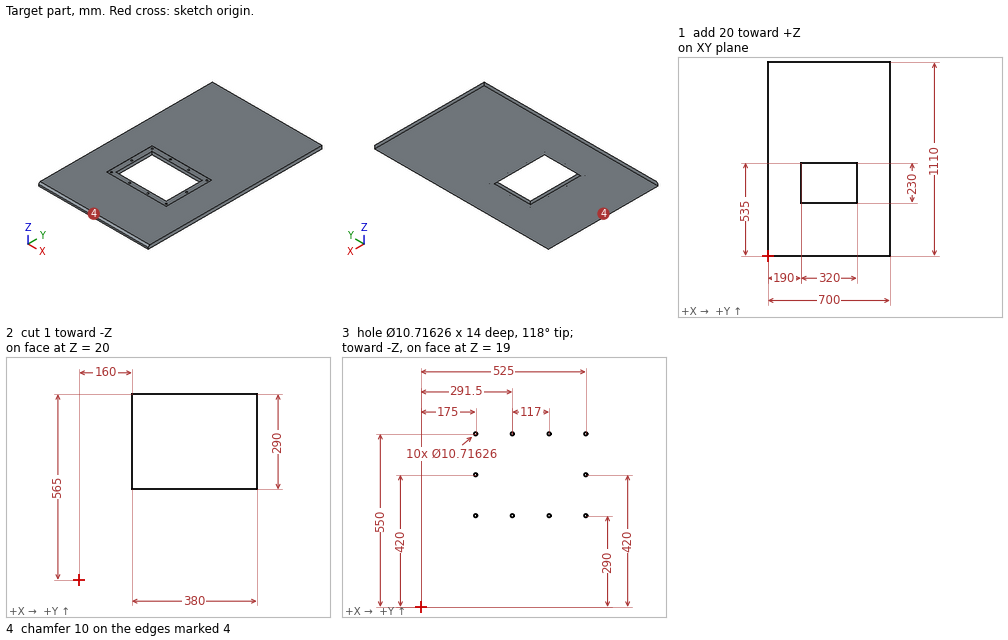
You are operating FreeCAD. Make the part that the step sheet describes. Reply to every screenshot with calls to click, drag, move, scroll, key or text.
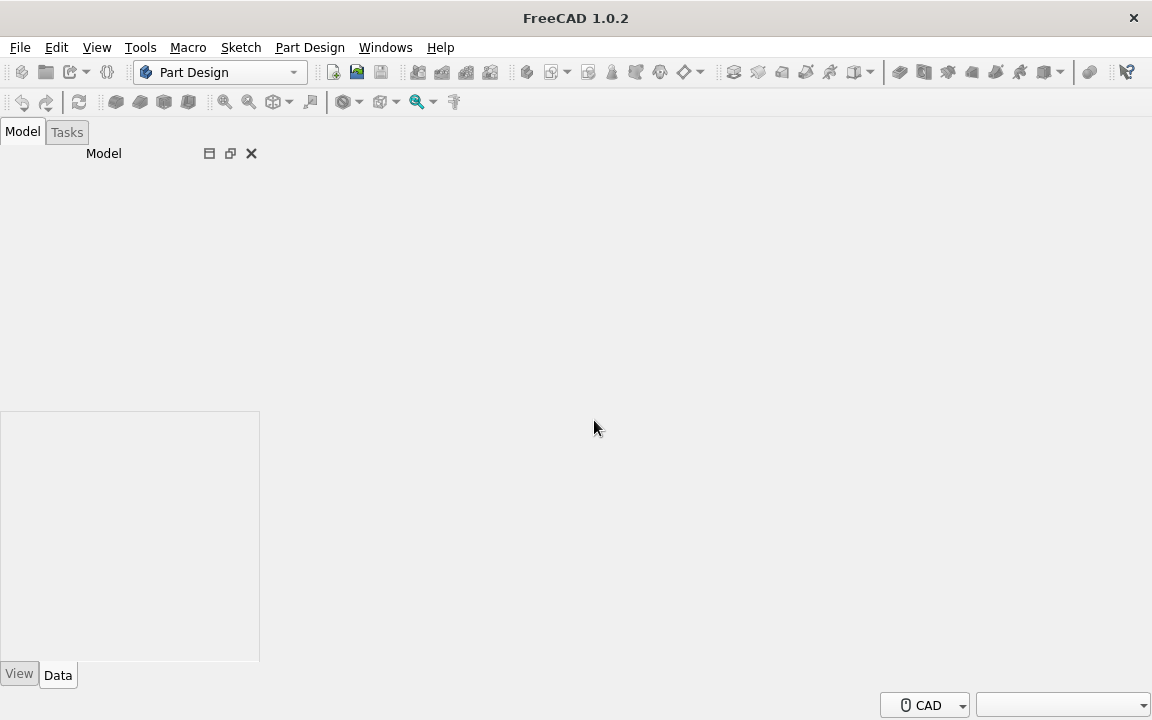
key(ctrl+n)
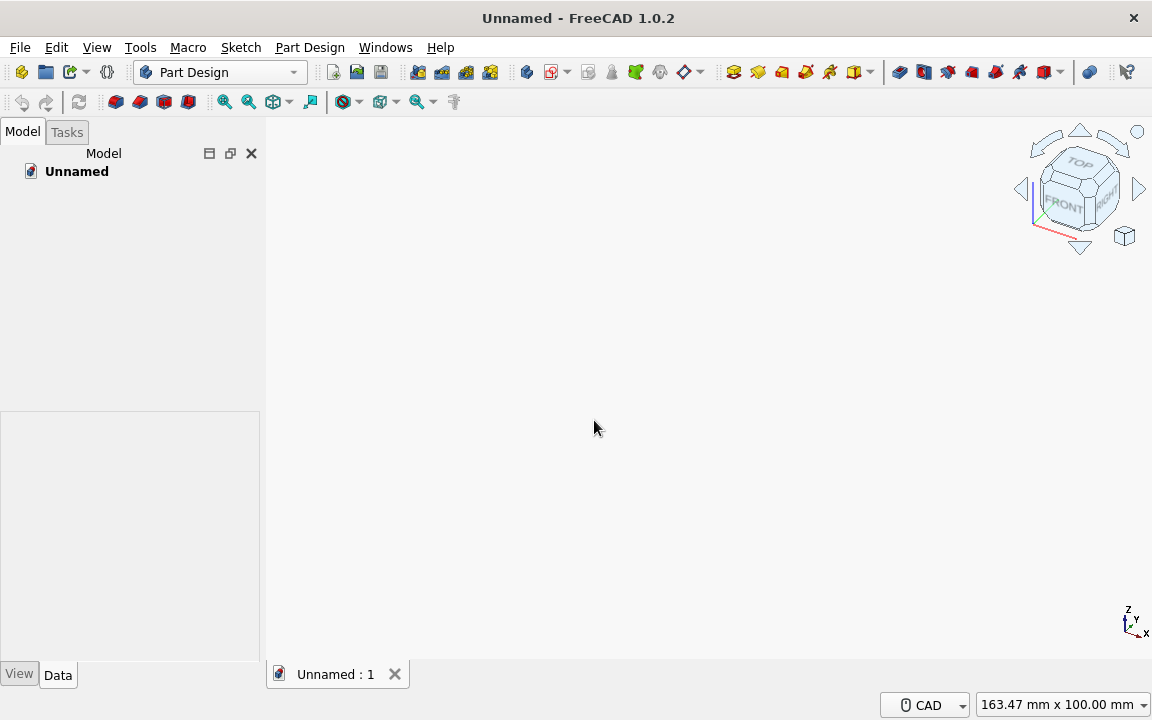
click(552, 72)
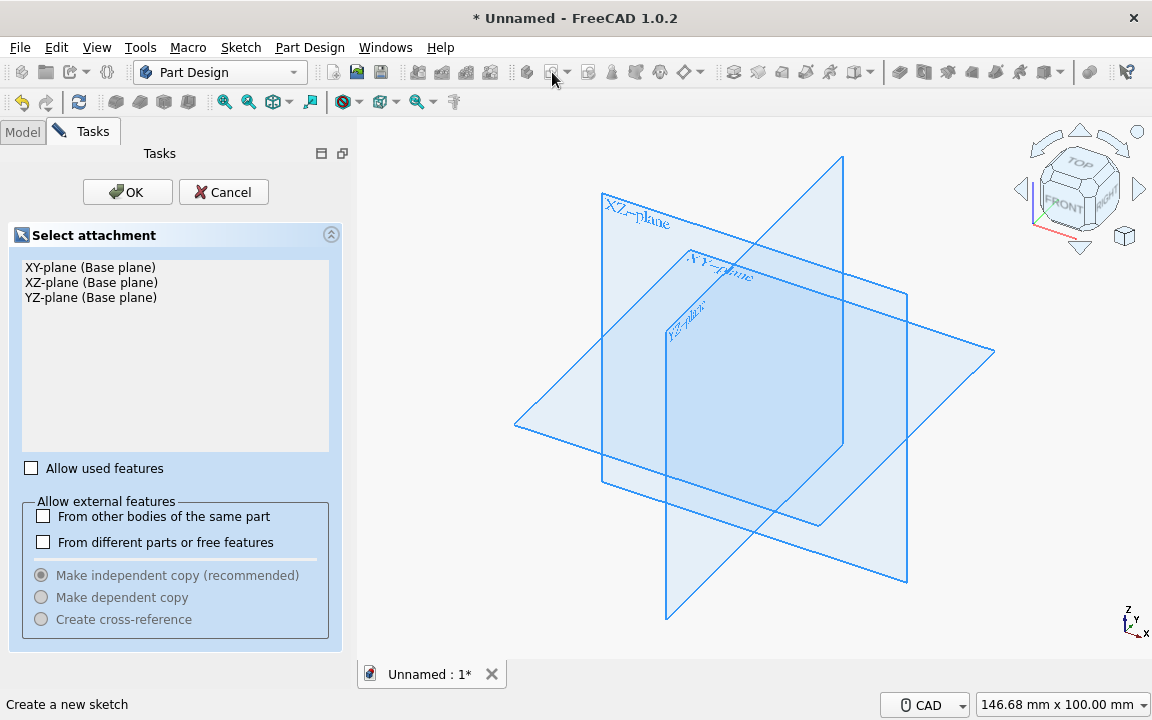
click(82, 268)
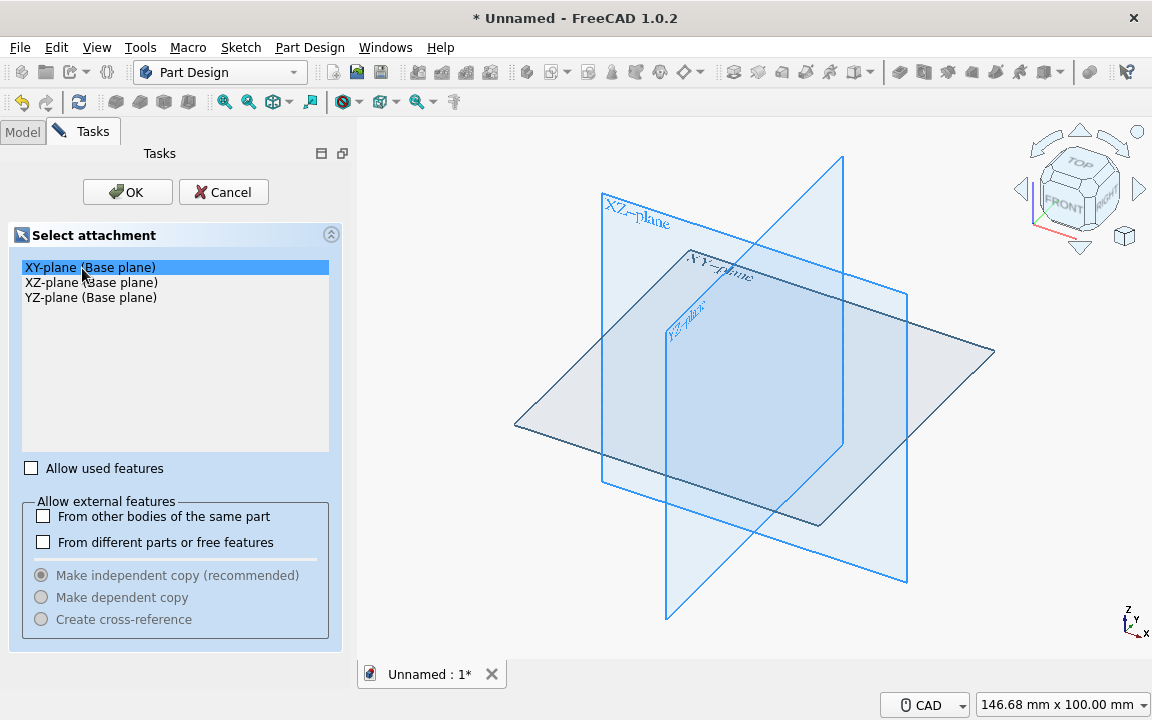
click(128, 192)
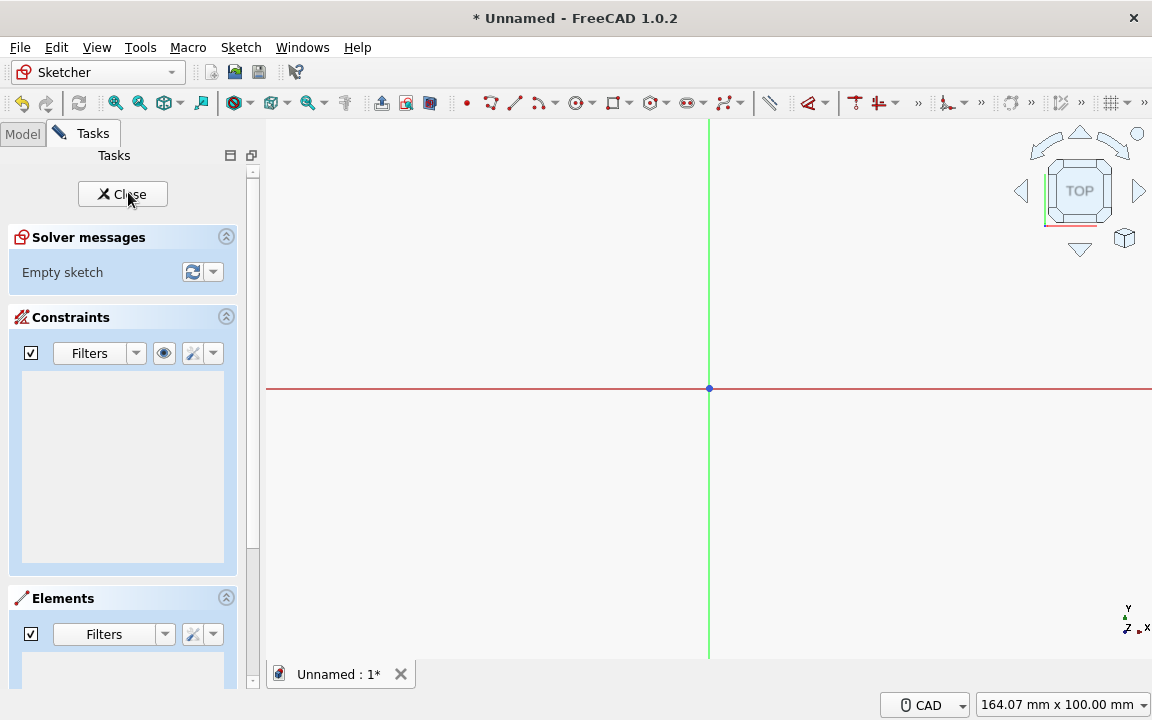
scroll(514, 583, down, 14)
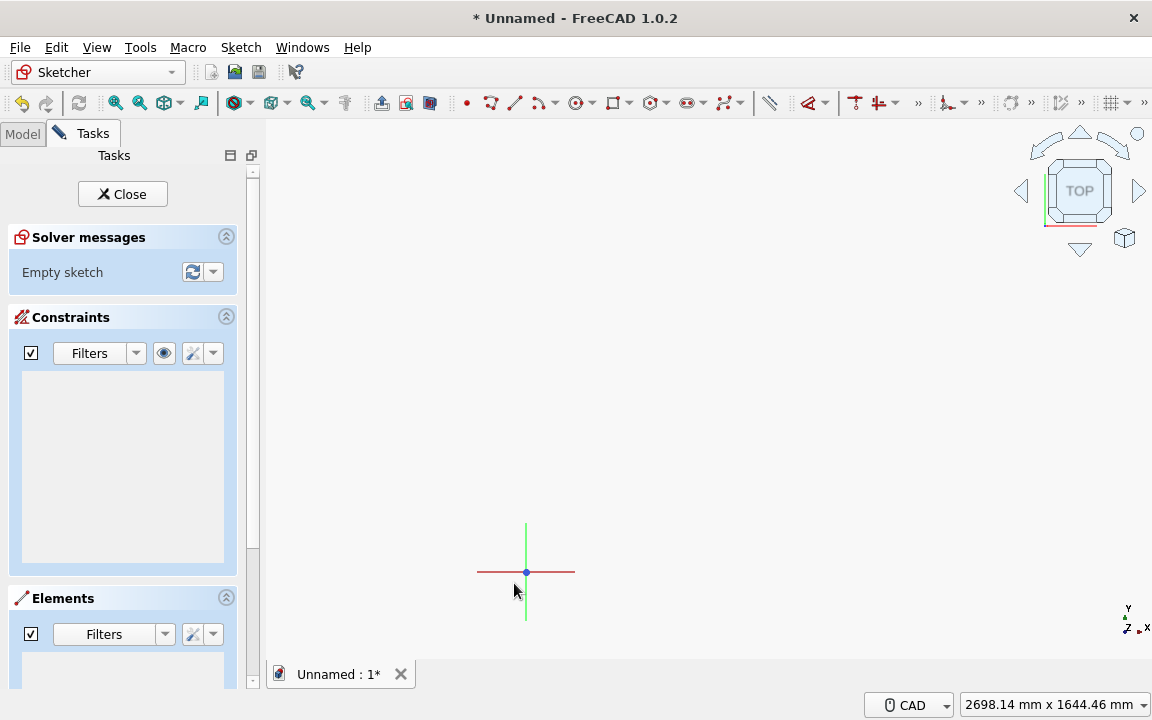
key(g)
key(r)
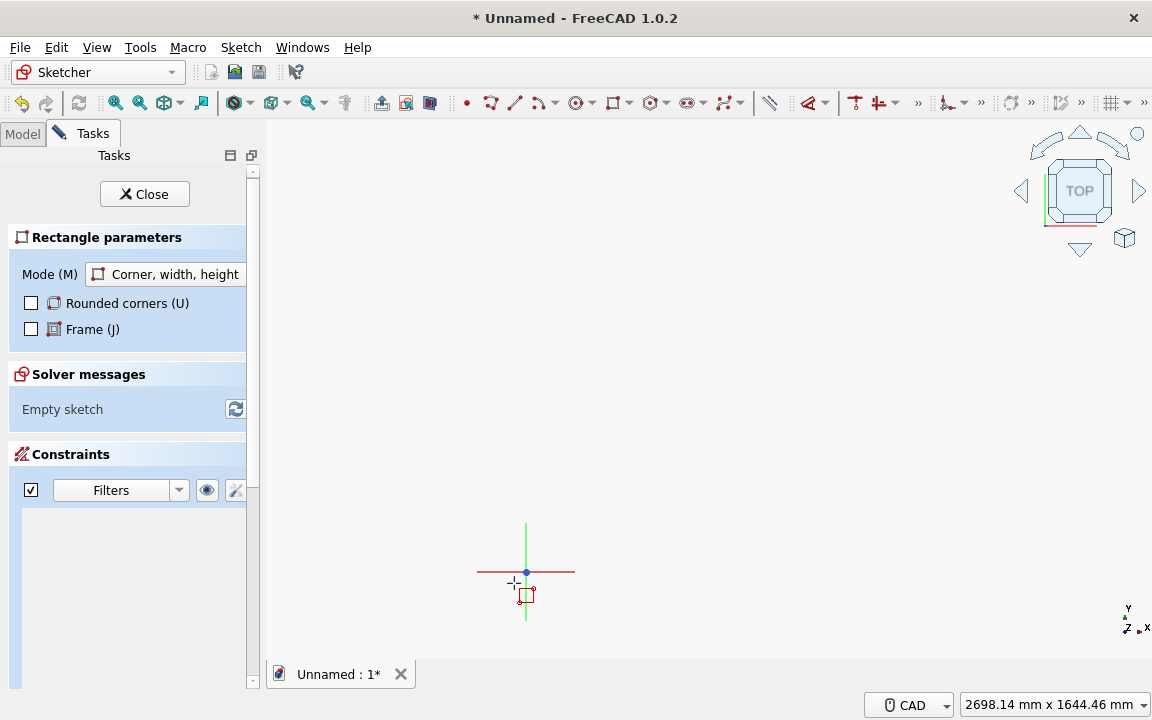
click(526, 572)
move(756, 208)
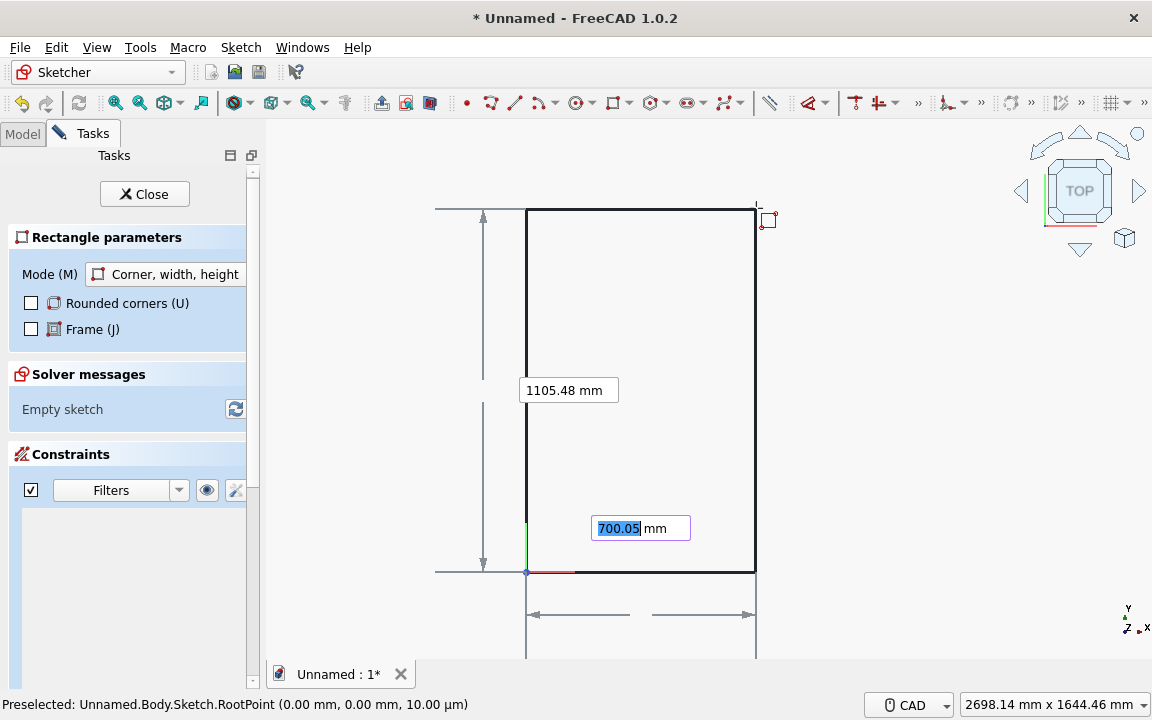
text(700)
key(Tab)
text(1110)
key(Return)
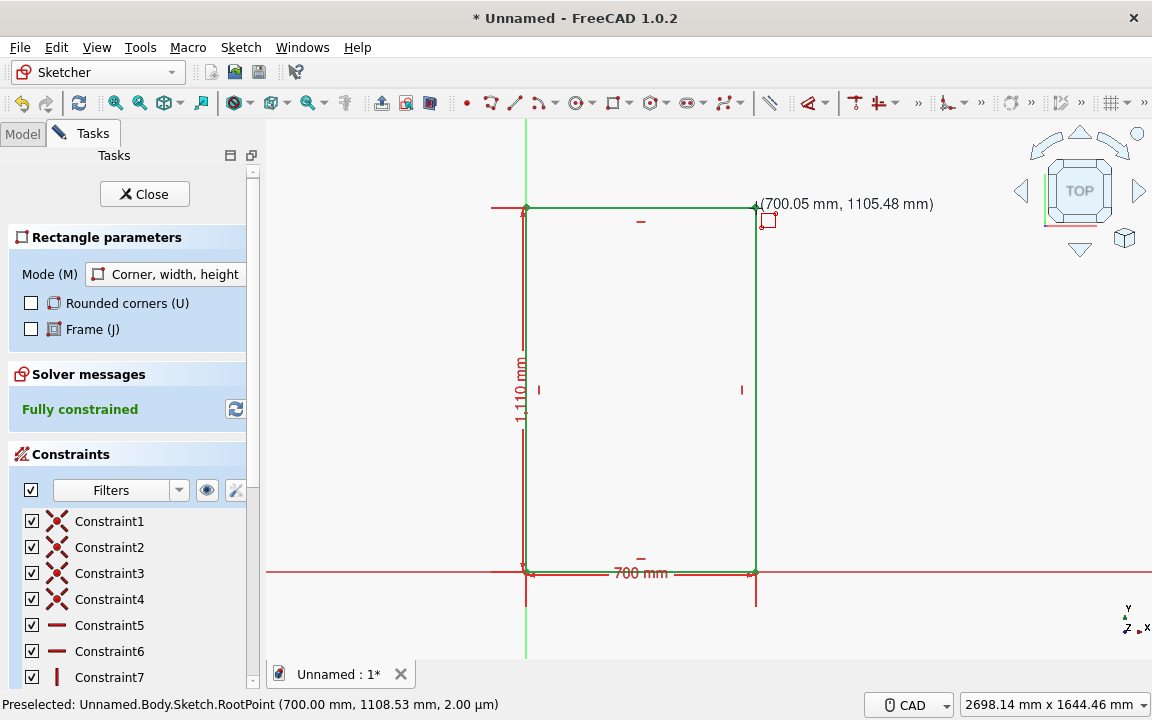
click(589, 396)
move(694, 472)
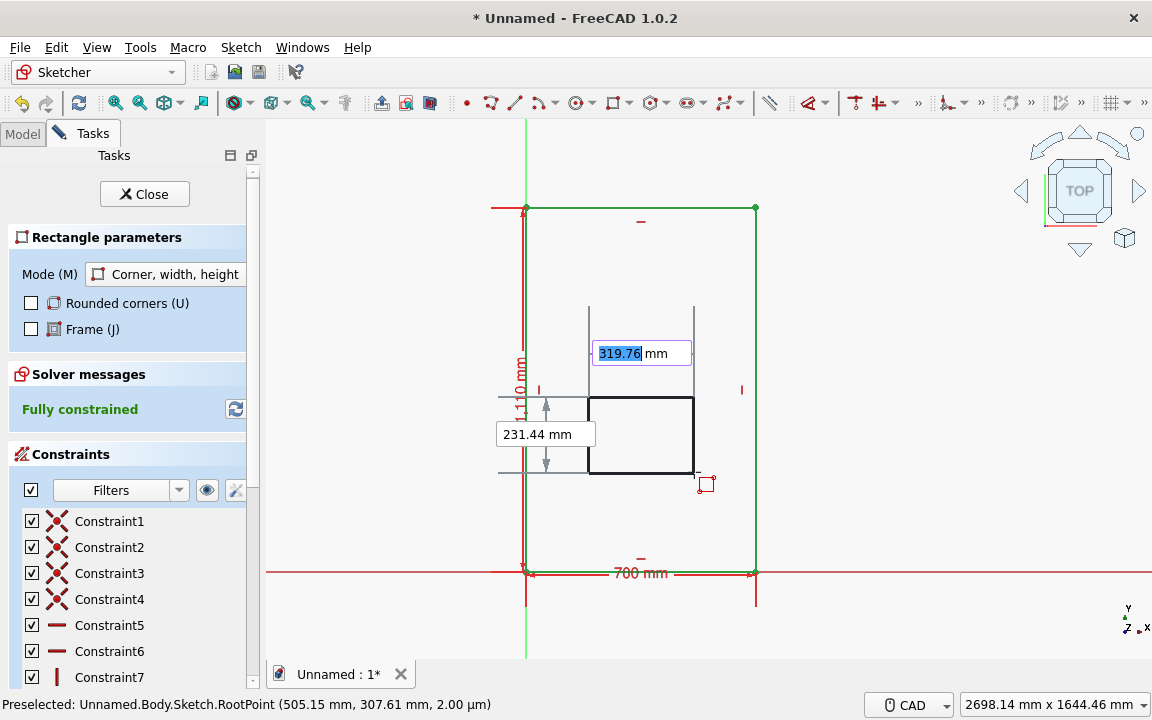
text(320)
key(Tab)
text(230)
key(Return)
key(Escape)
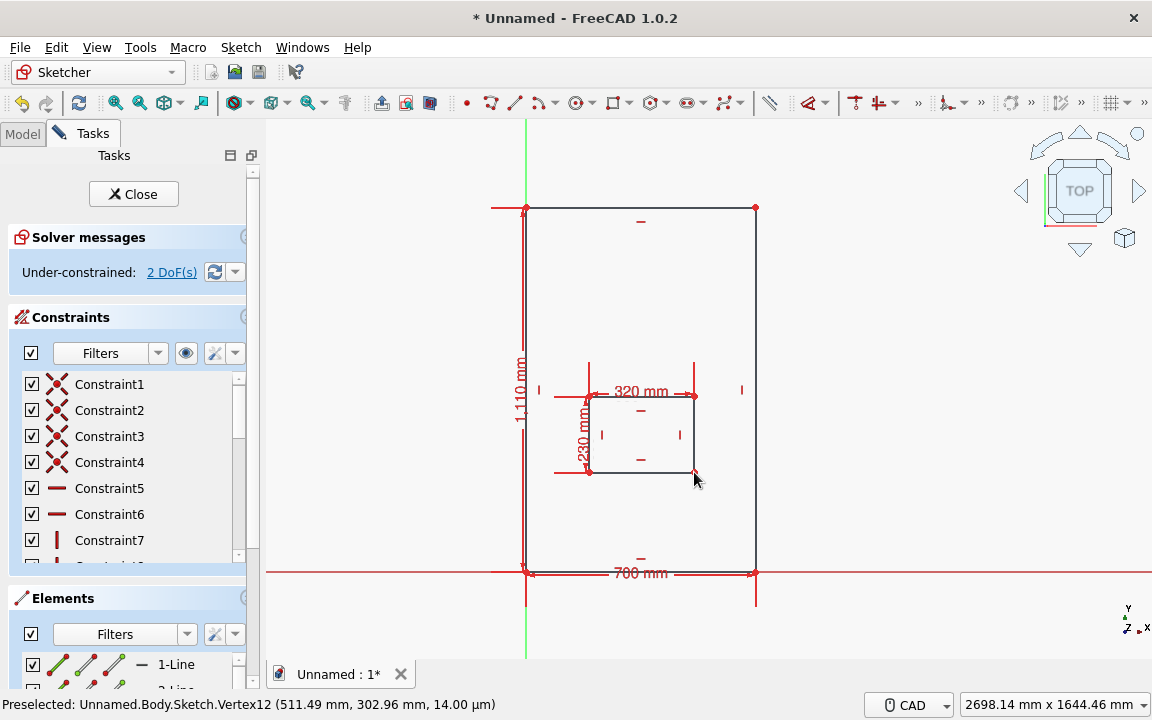
key(d)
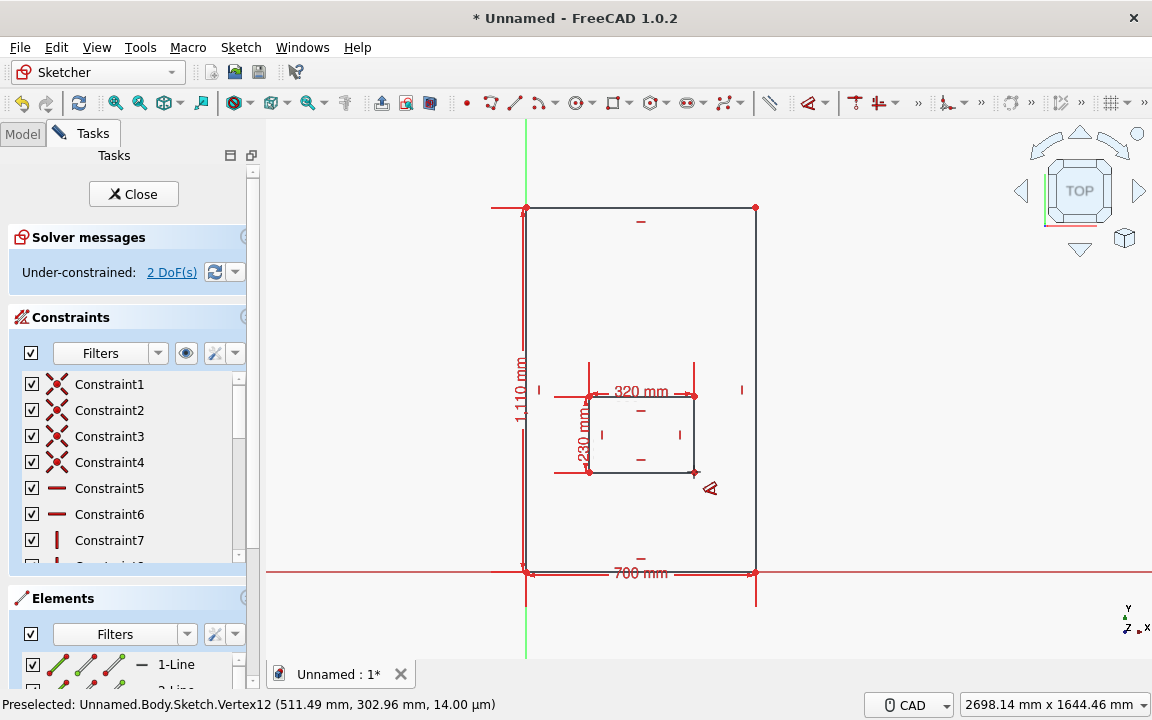
click(589, 397)
click(558, 606)